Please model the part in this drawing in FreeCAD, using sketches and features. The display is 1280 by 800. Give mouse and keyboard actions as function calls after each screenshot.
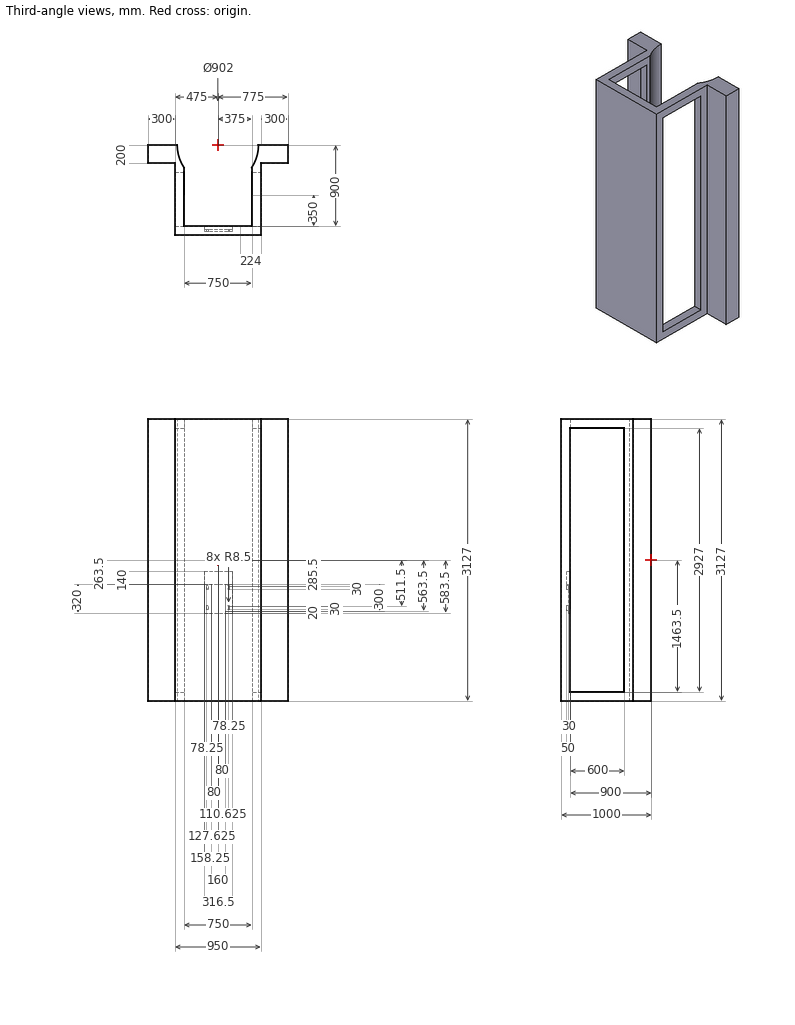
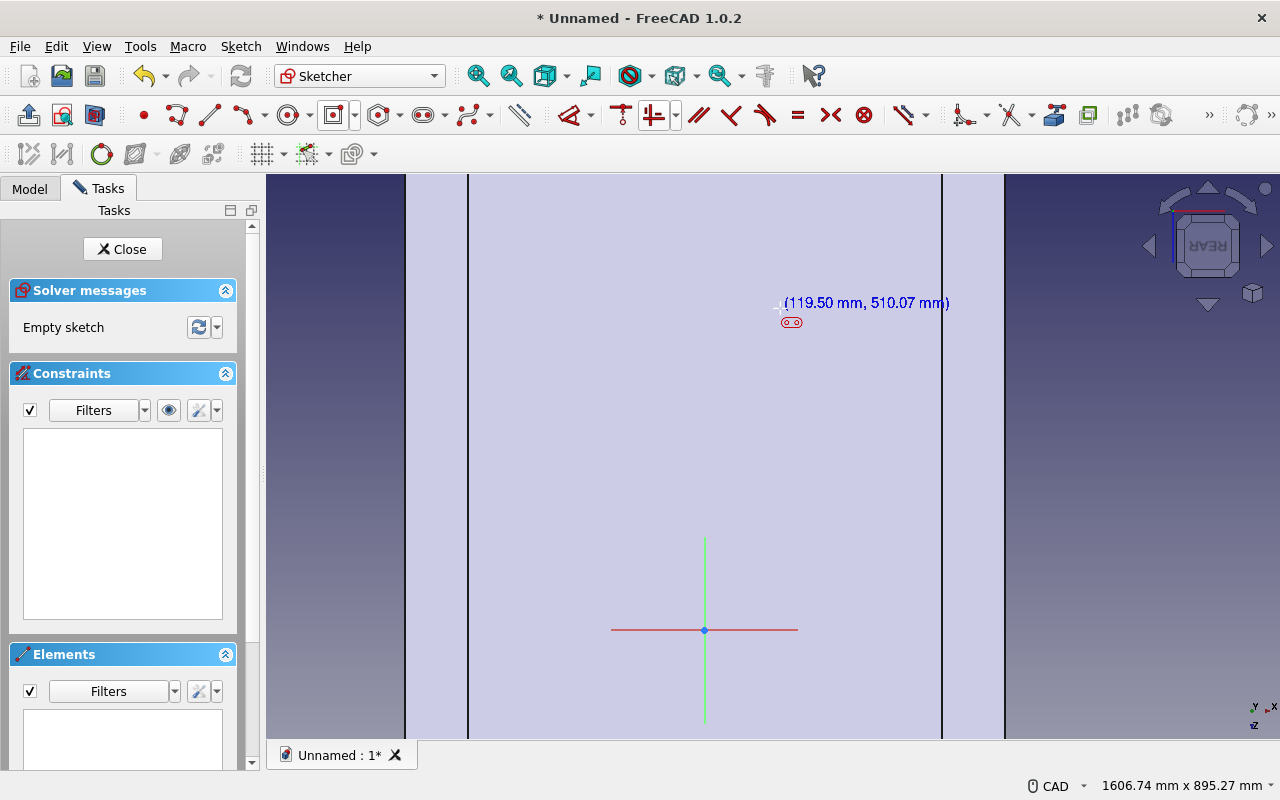
click(780, 307)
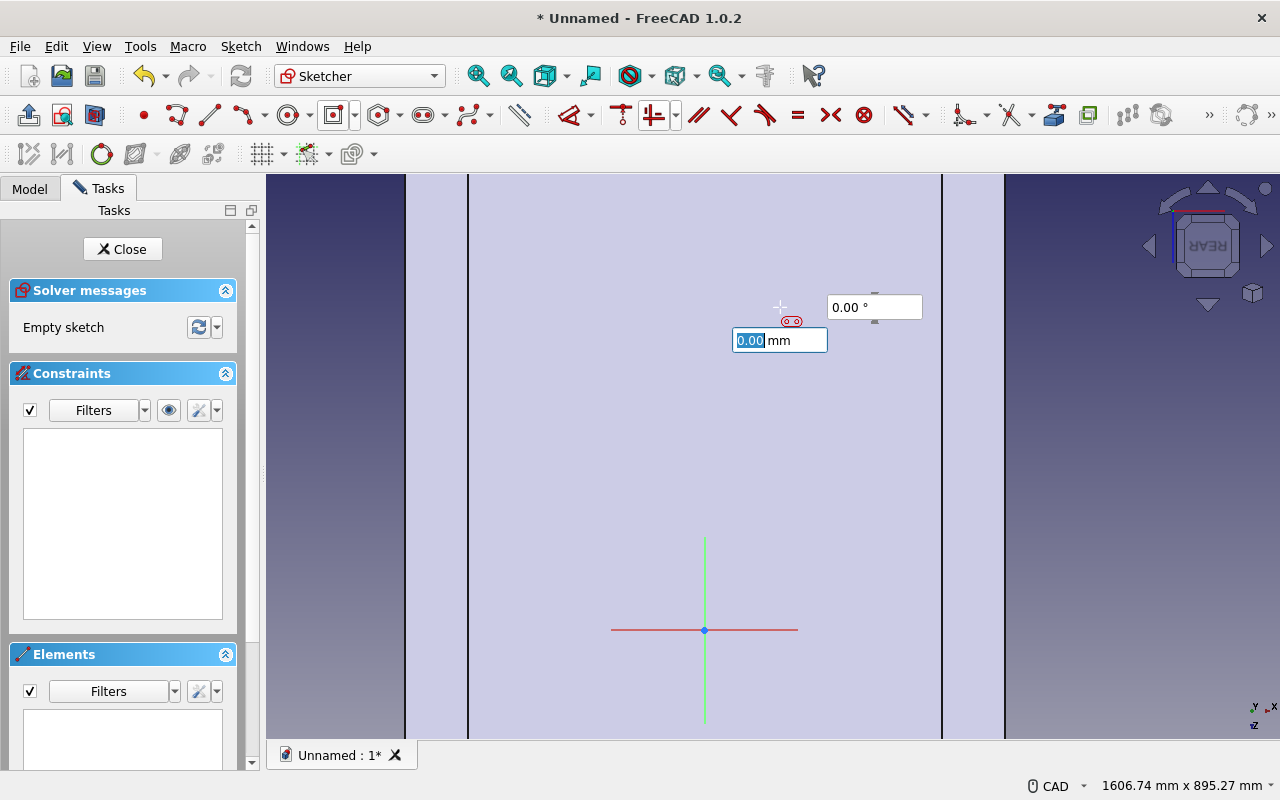
click(780, 289)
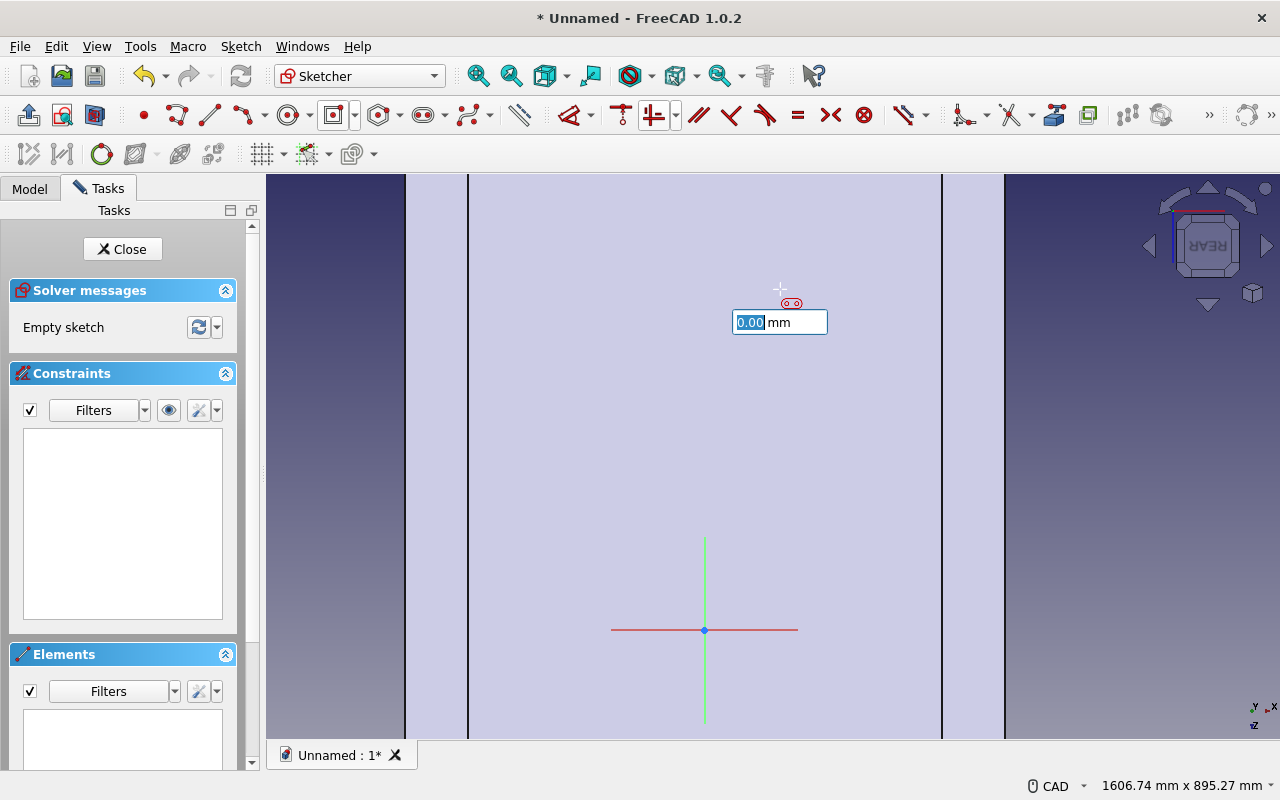
scroll(775, 298, up, 6)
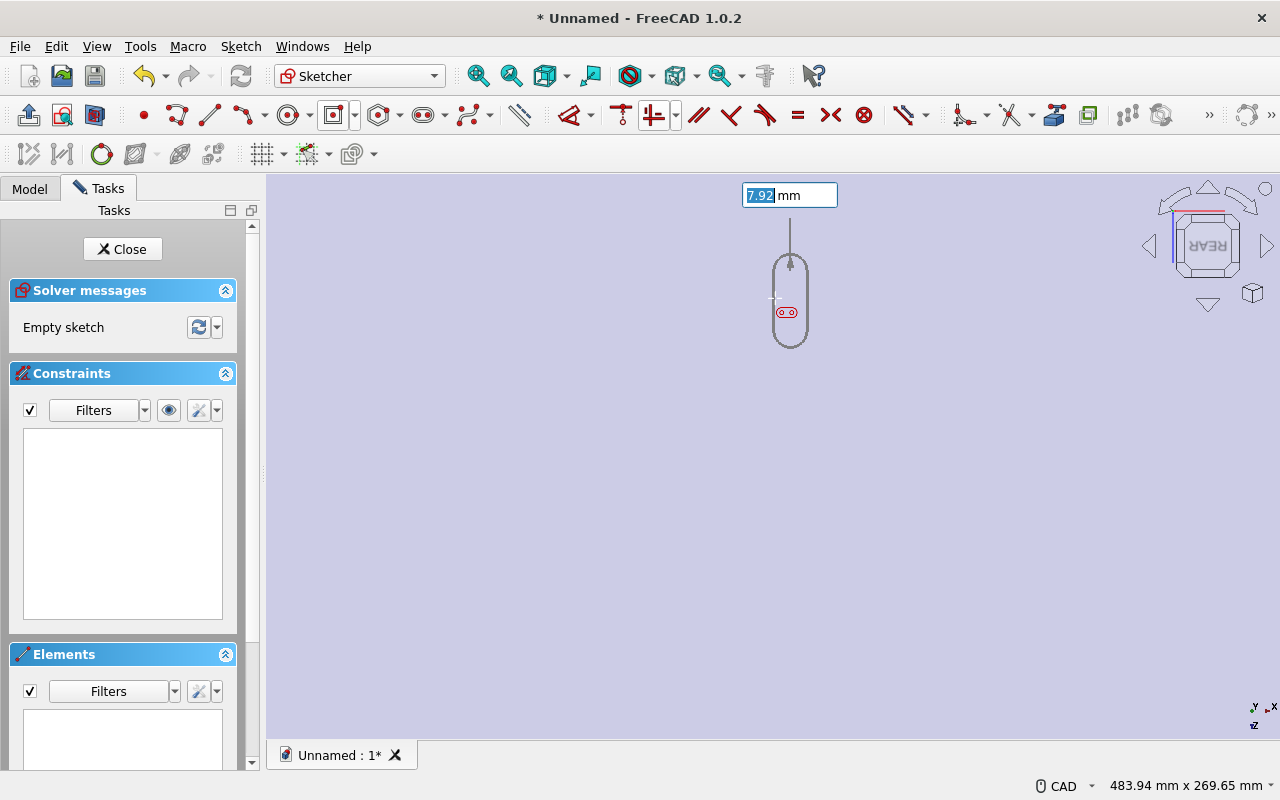
click(773, 298)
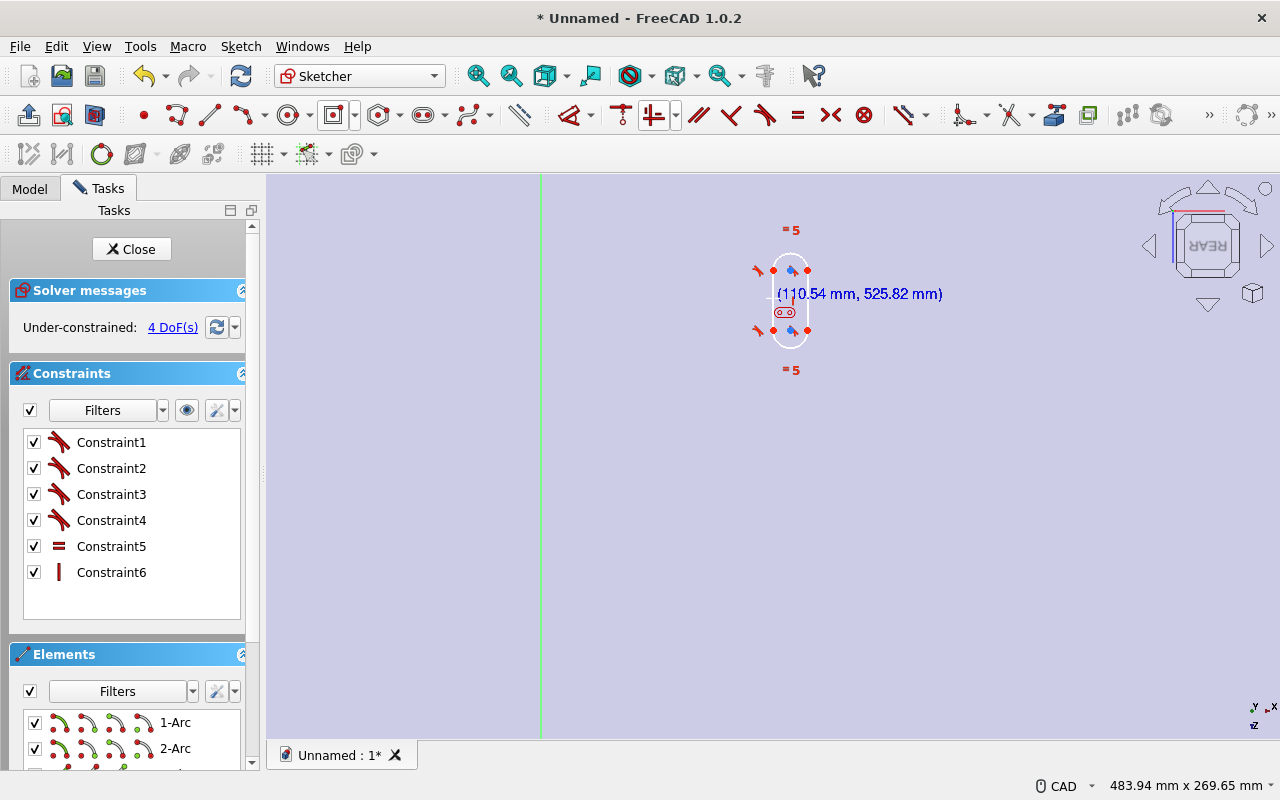
scroll(775, 298, down, 6)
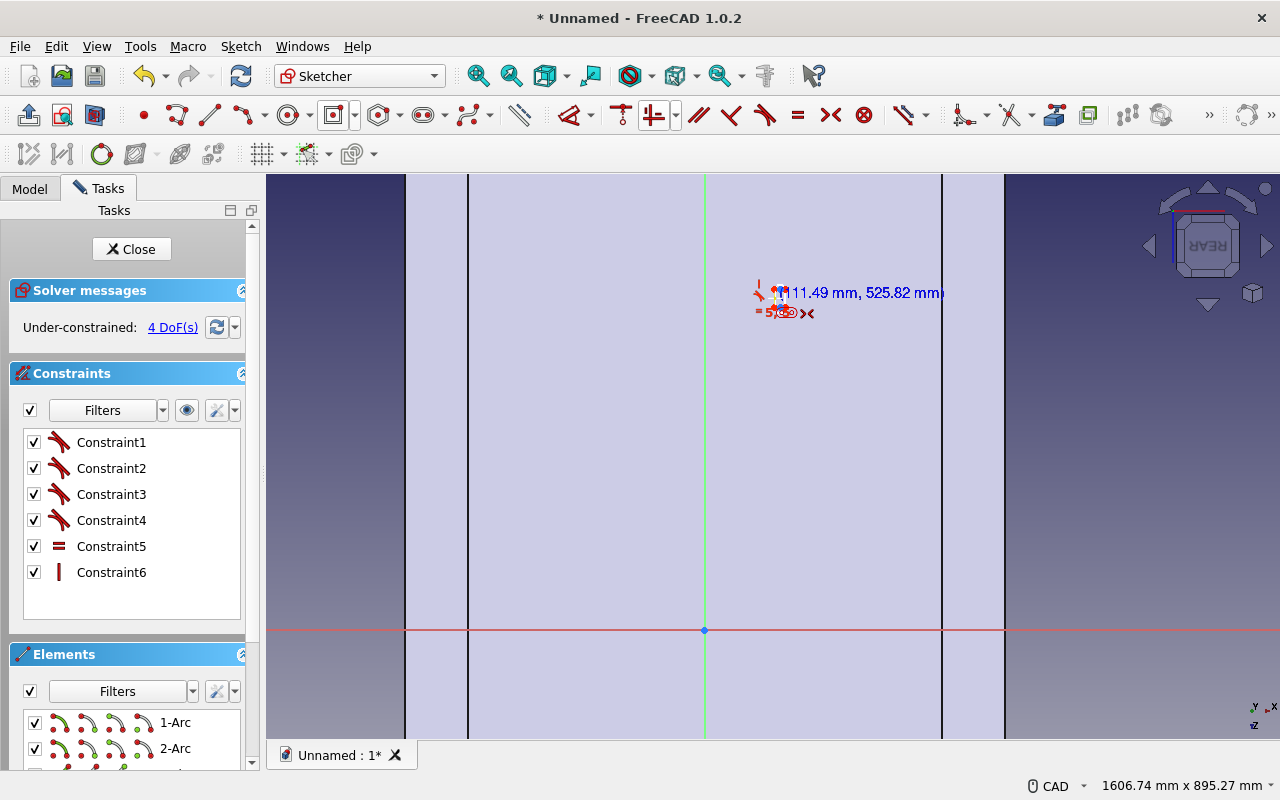
scroll(780, 450, up, 8)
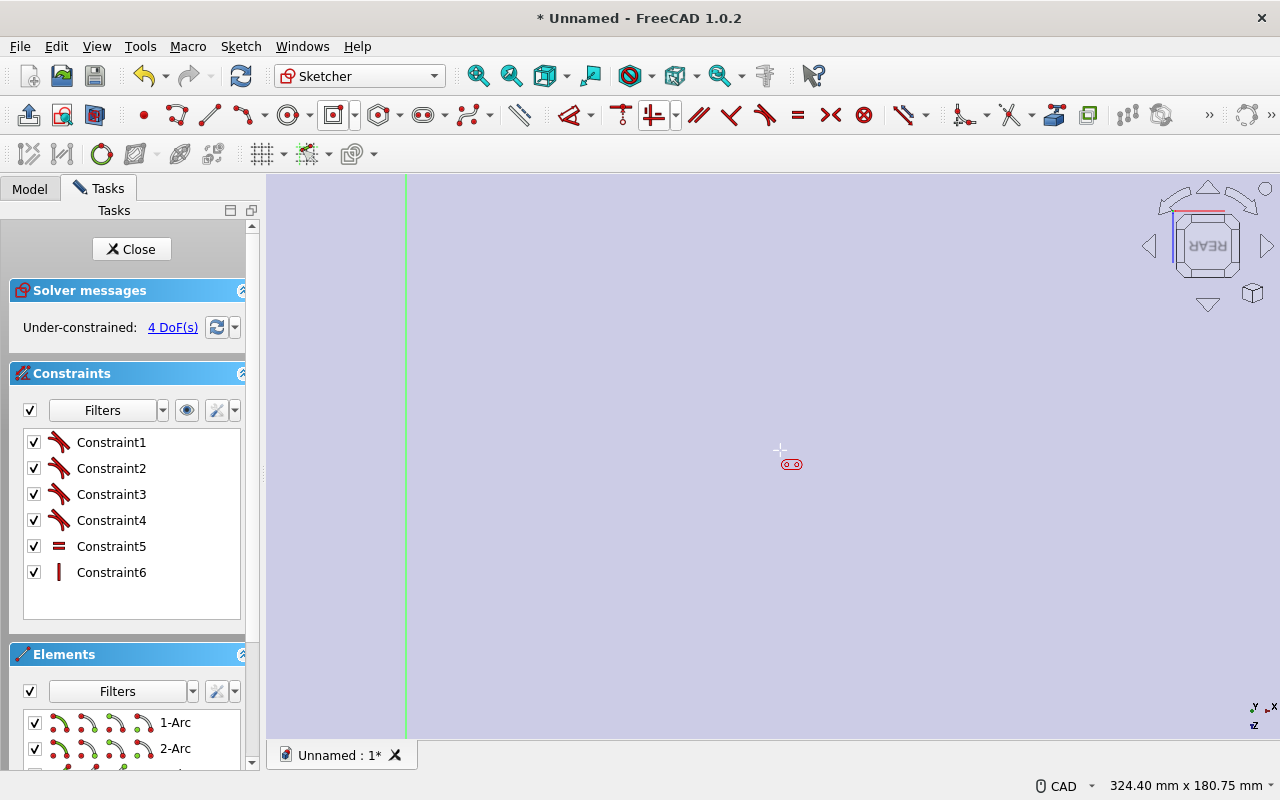
scroll(780, 450, down, 8)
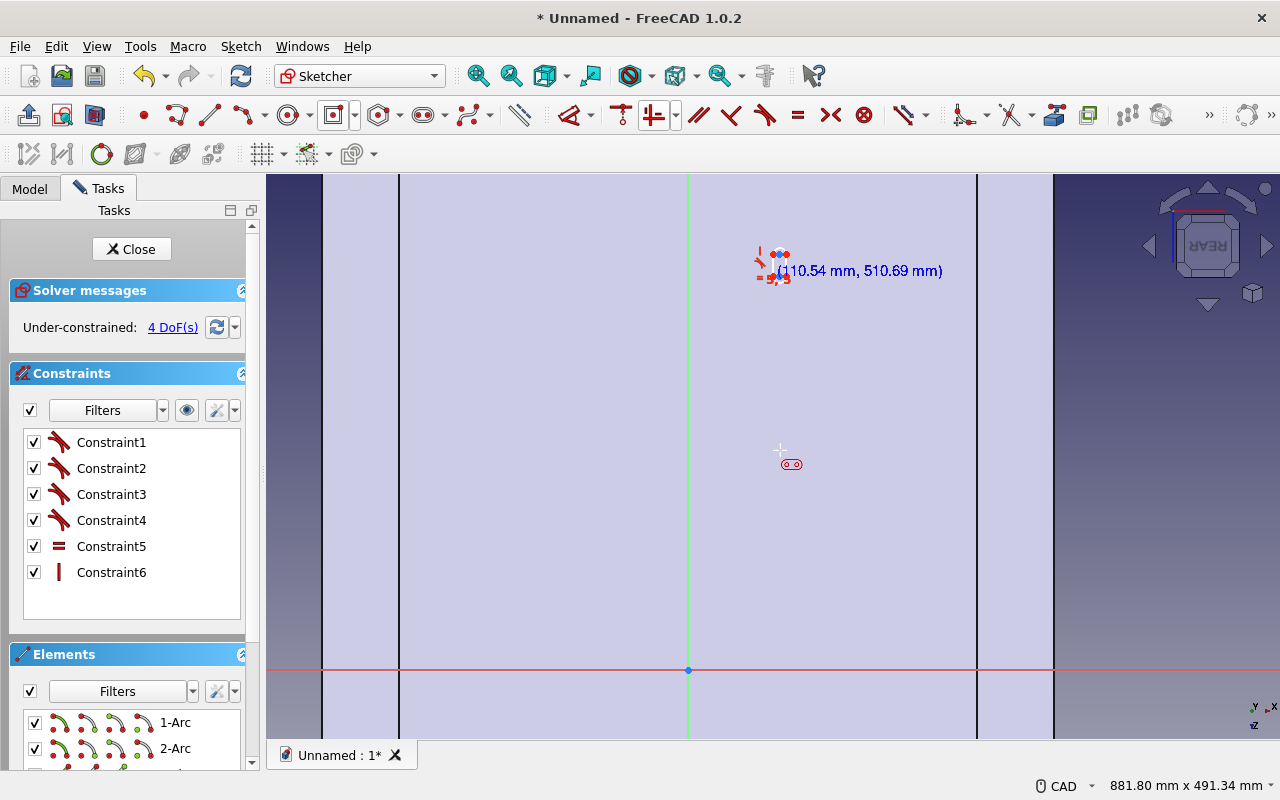
click(780, 450)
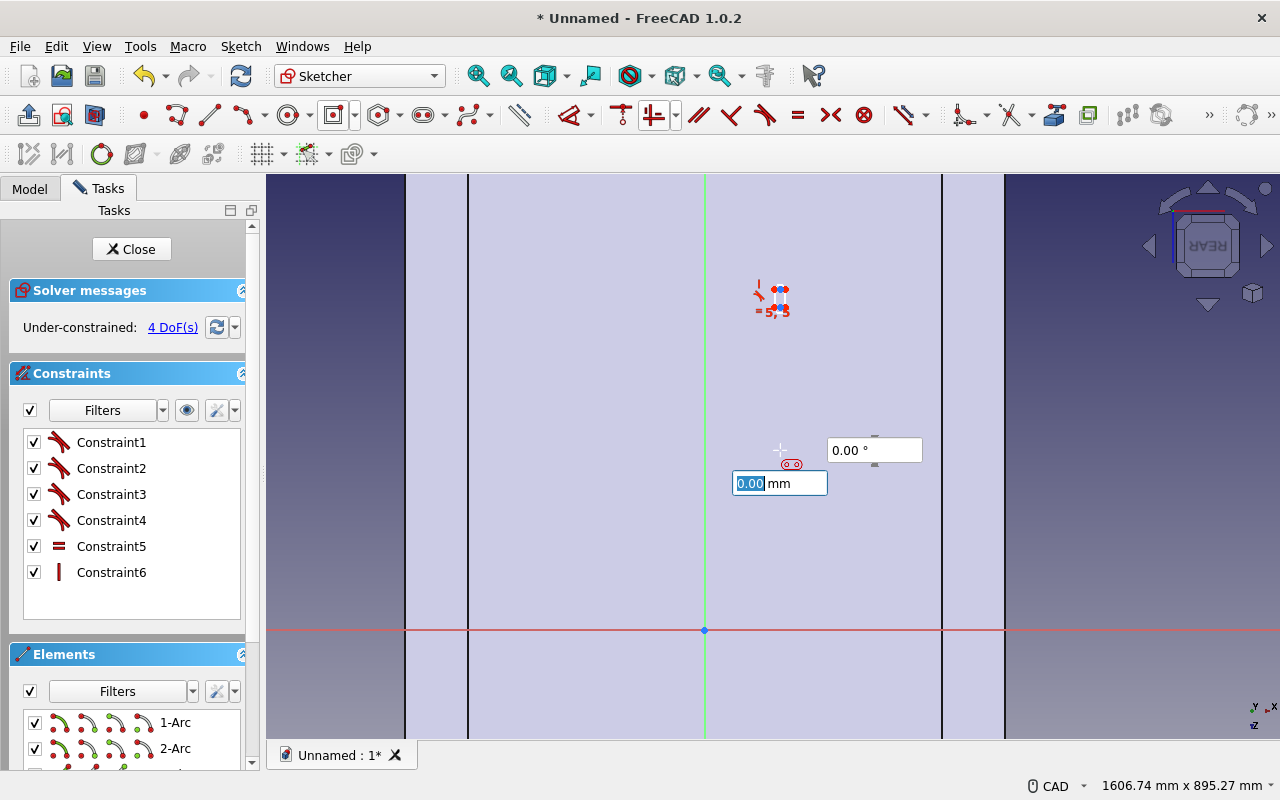
click(780, 431)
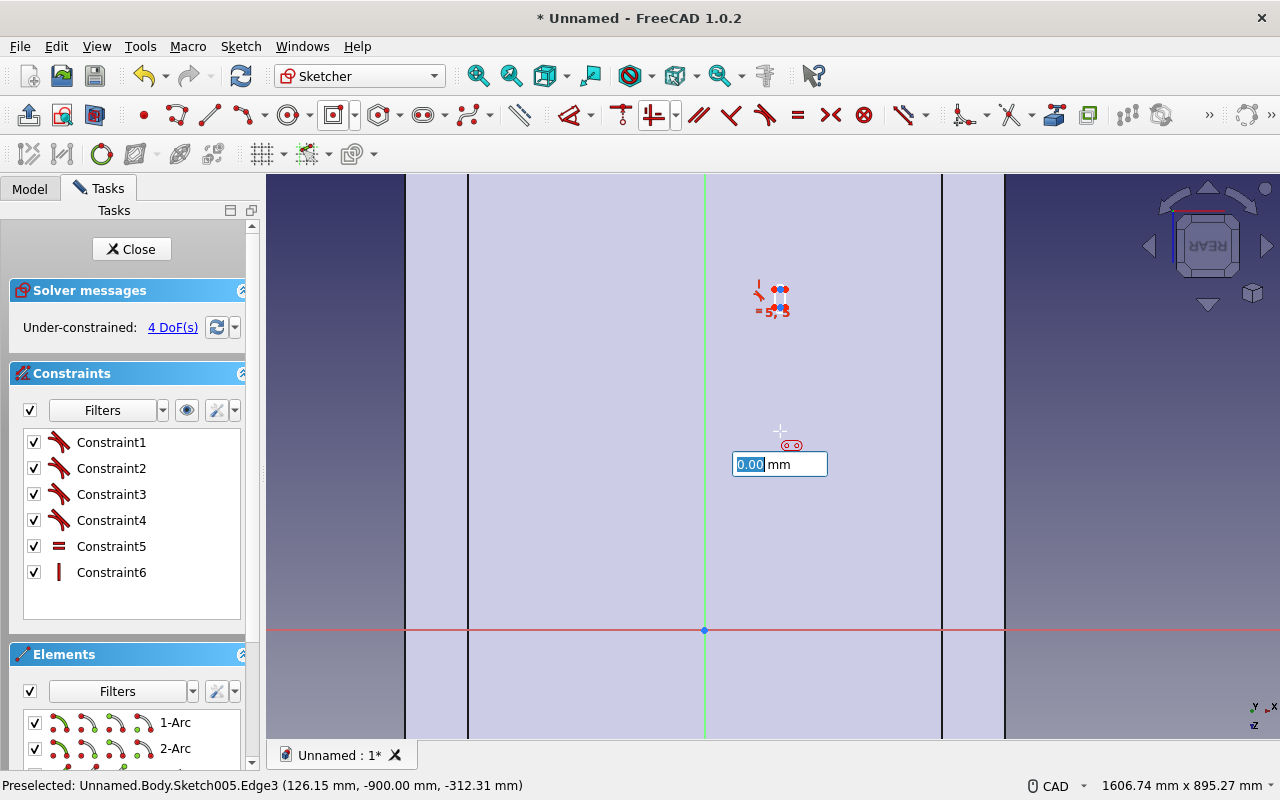
scroll(786, 441, up, 6)